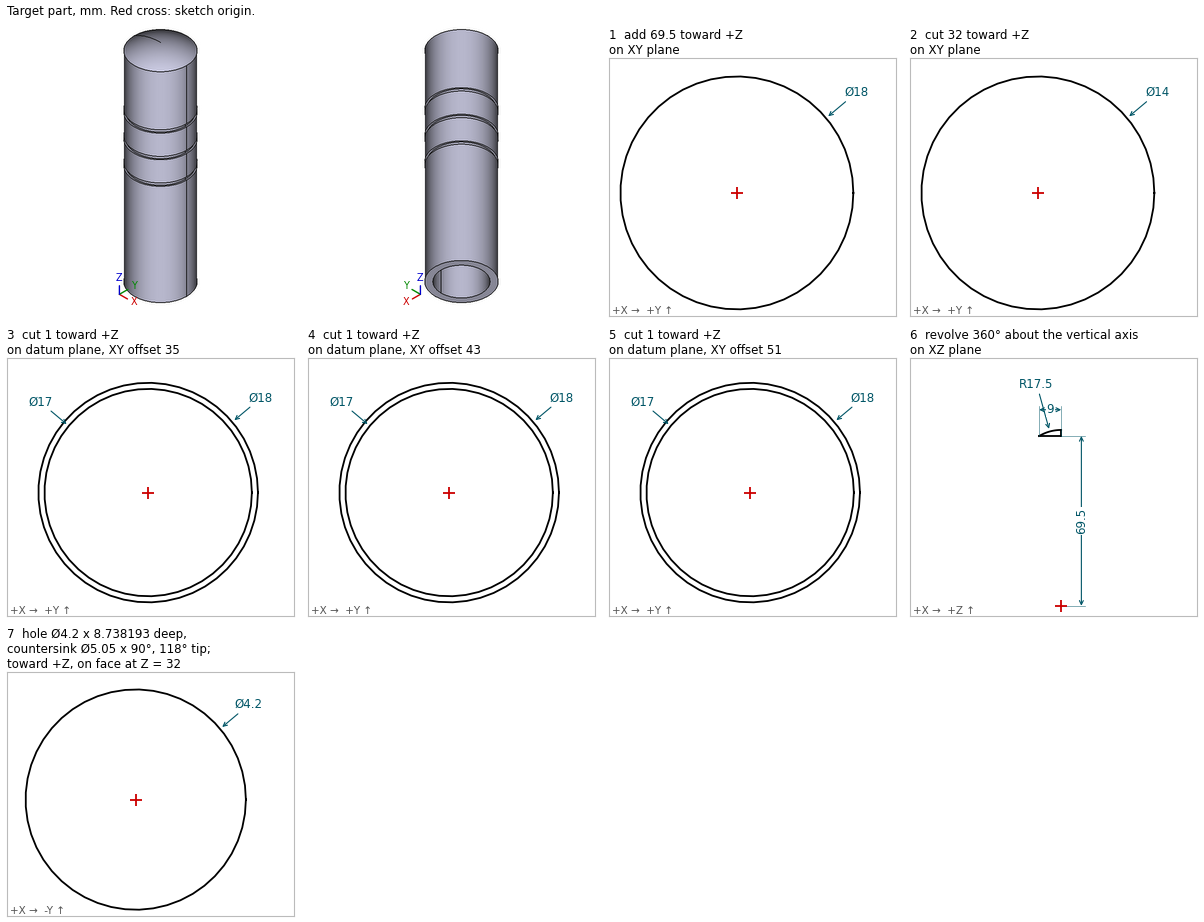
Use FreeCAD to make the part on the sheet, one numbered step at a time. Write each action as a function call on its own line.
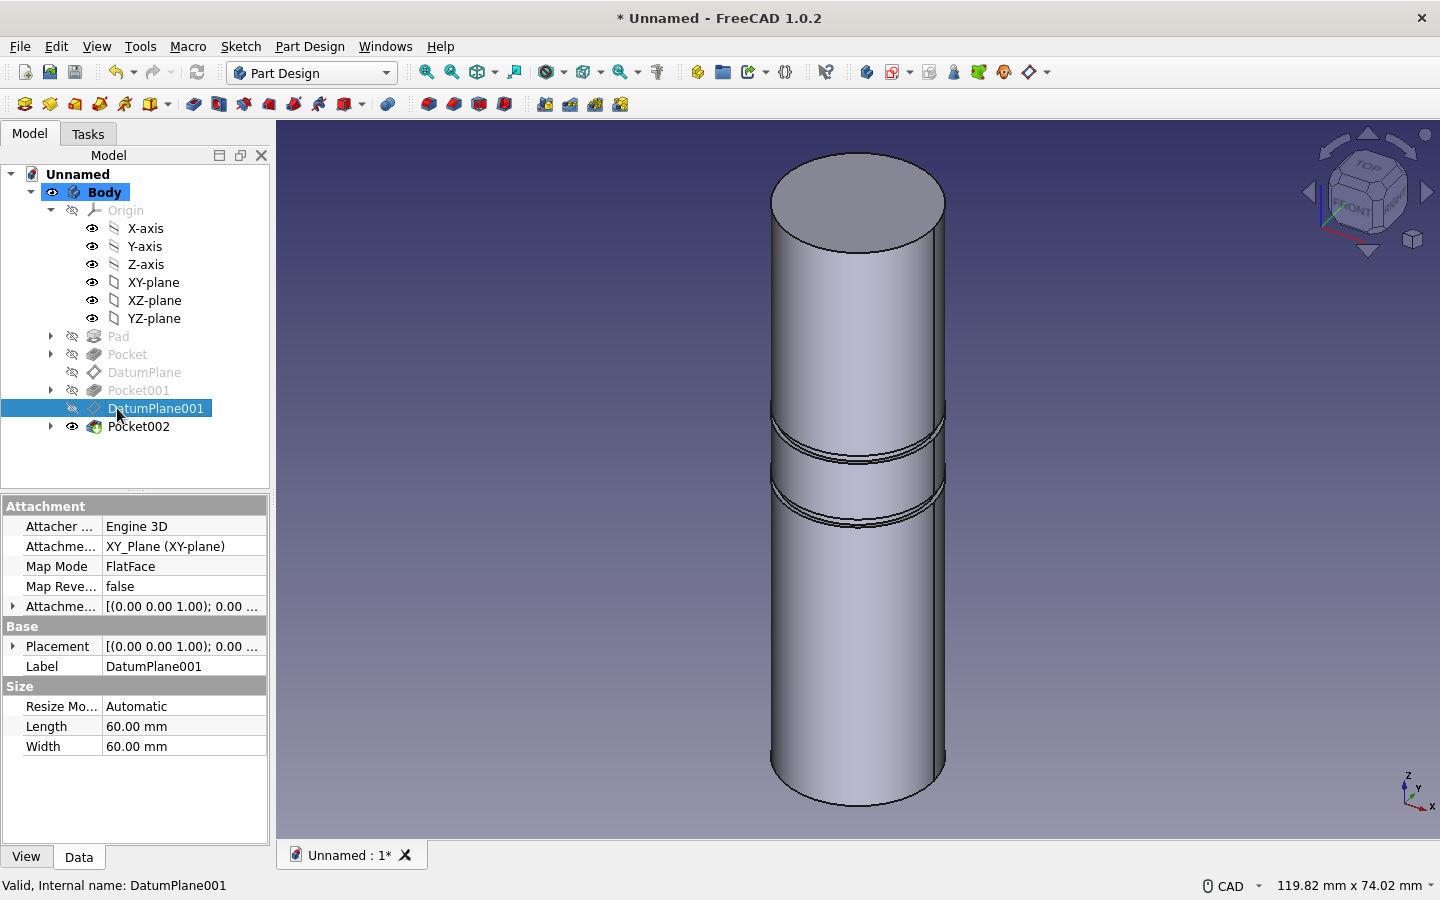
click(137, 282)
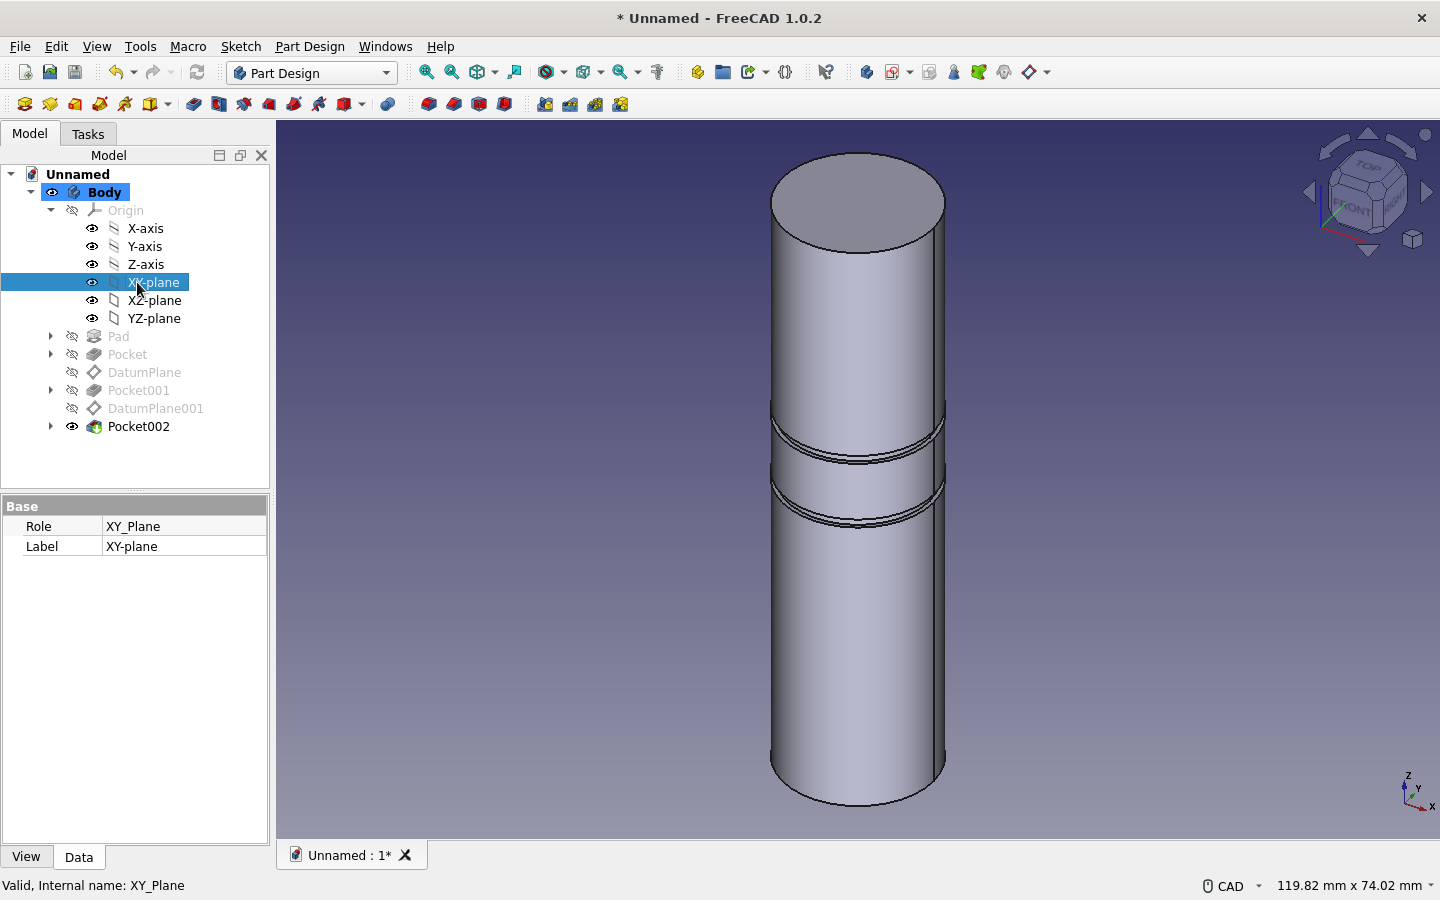
click(1028, 72)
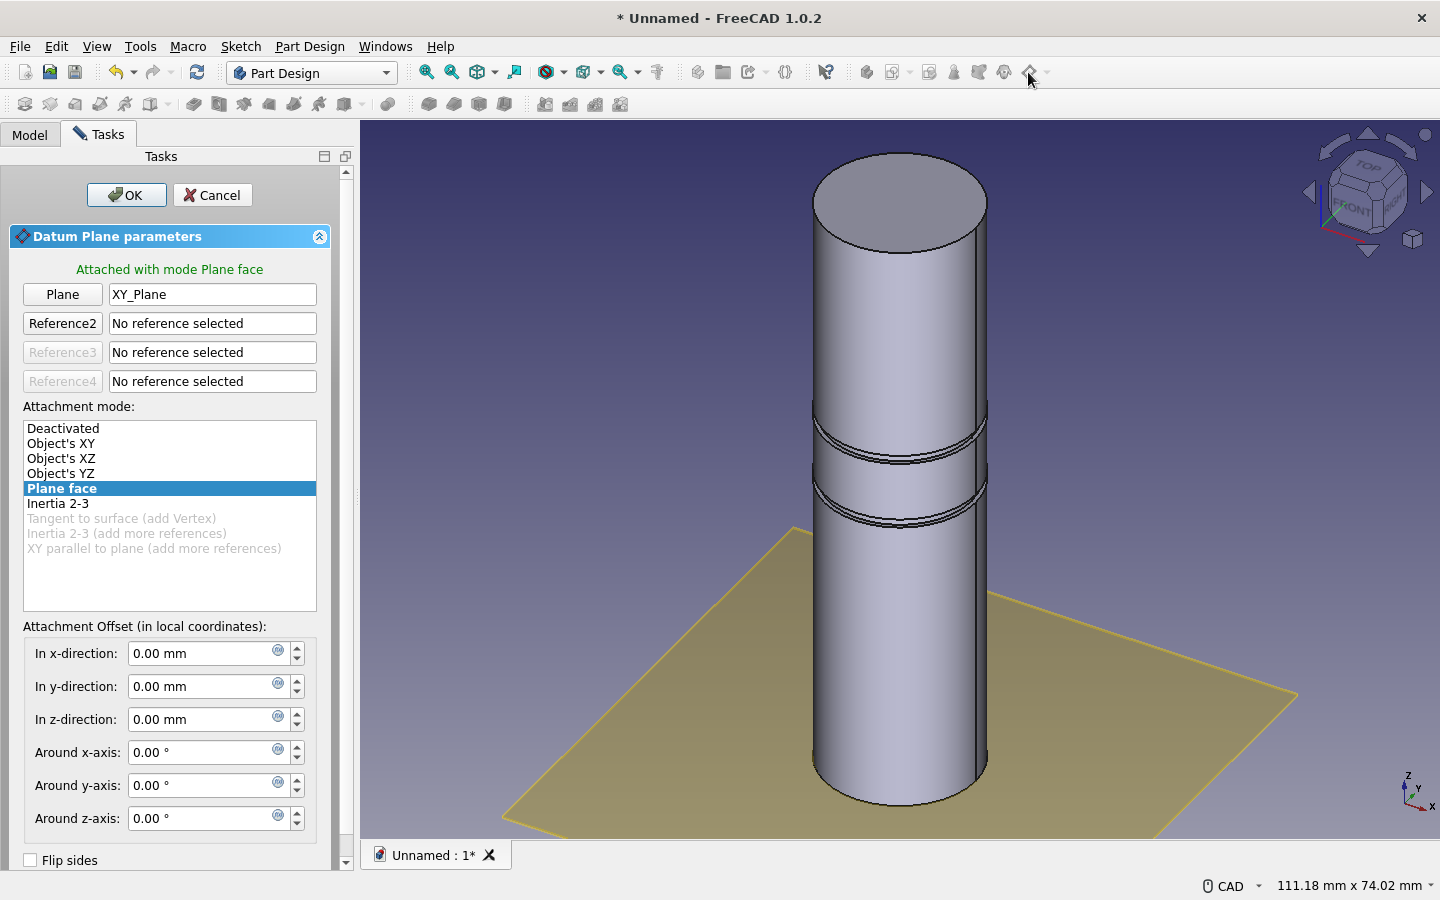
triple_click(210, 720)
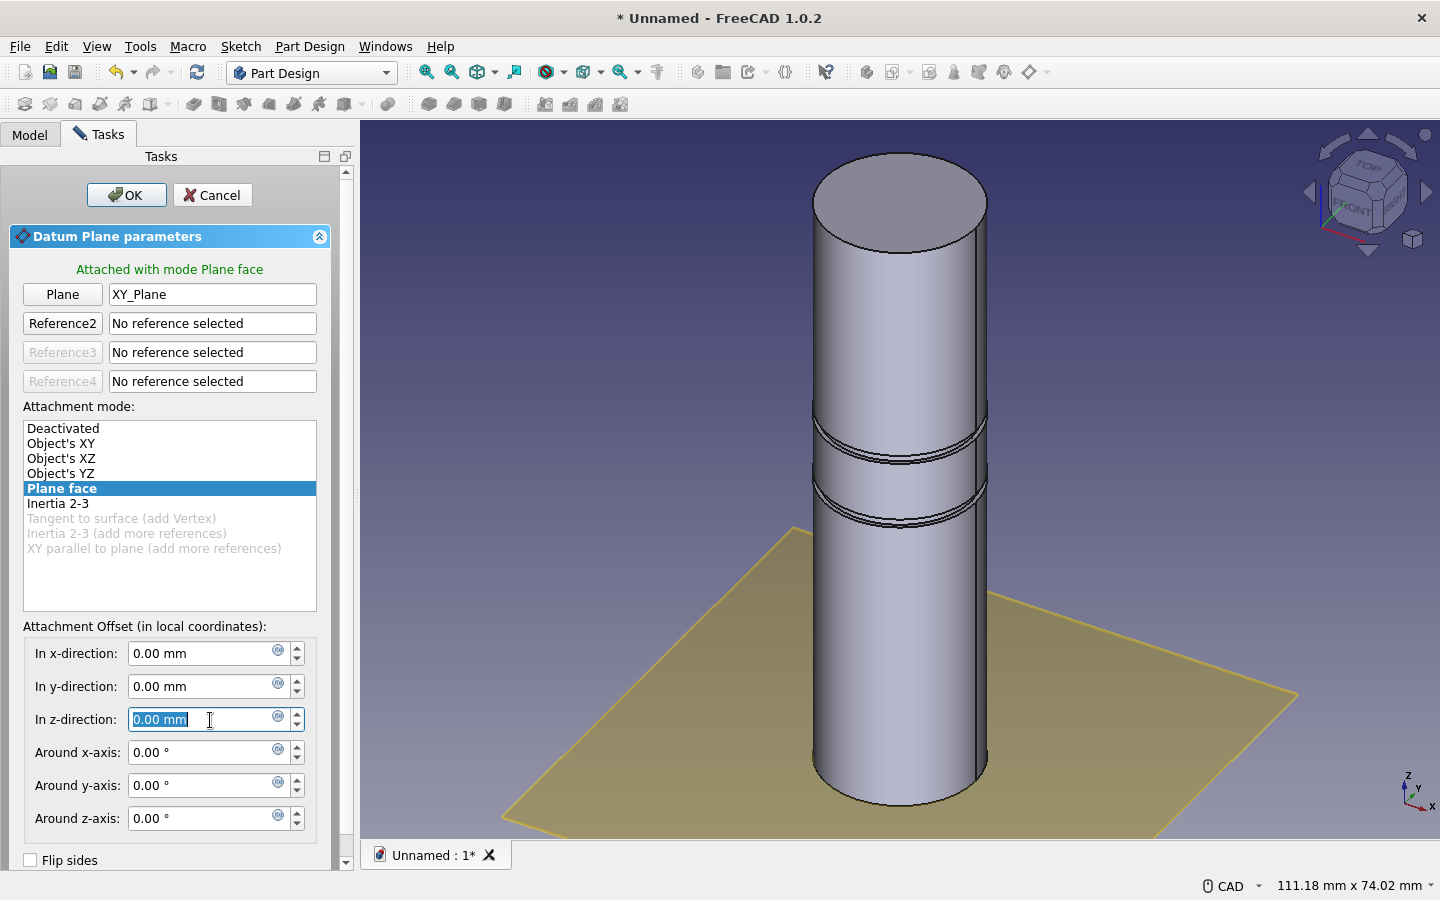
text(51)
key(Tab)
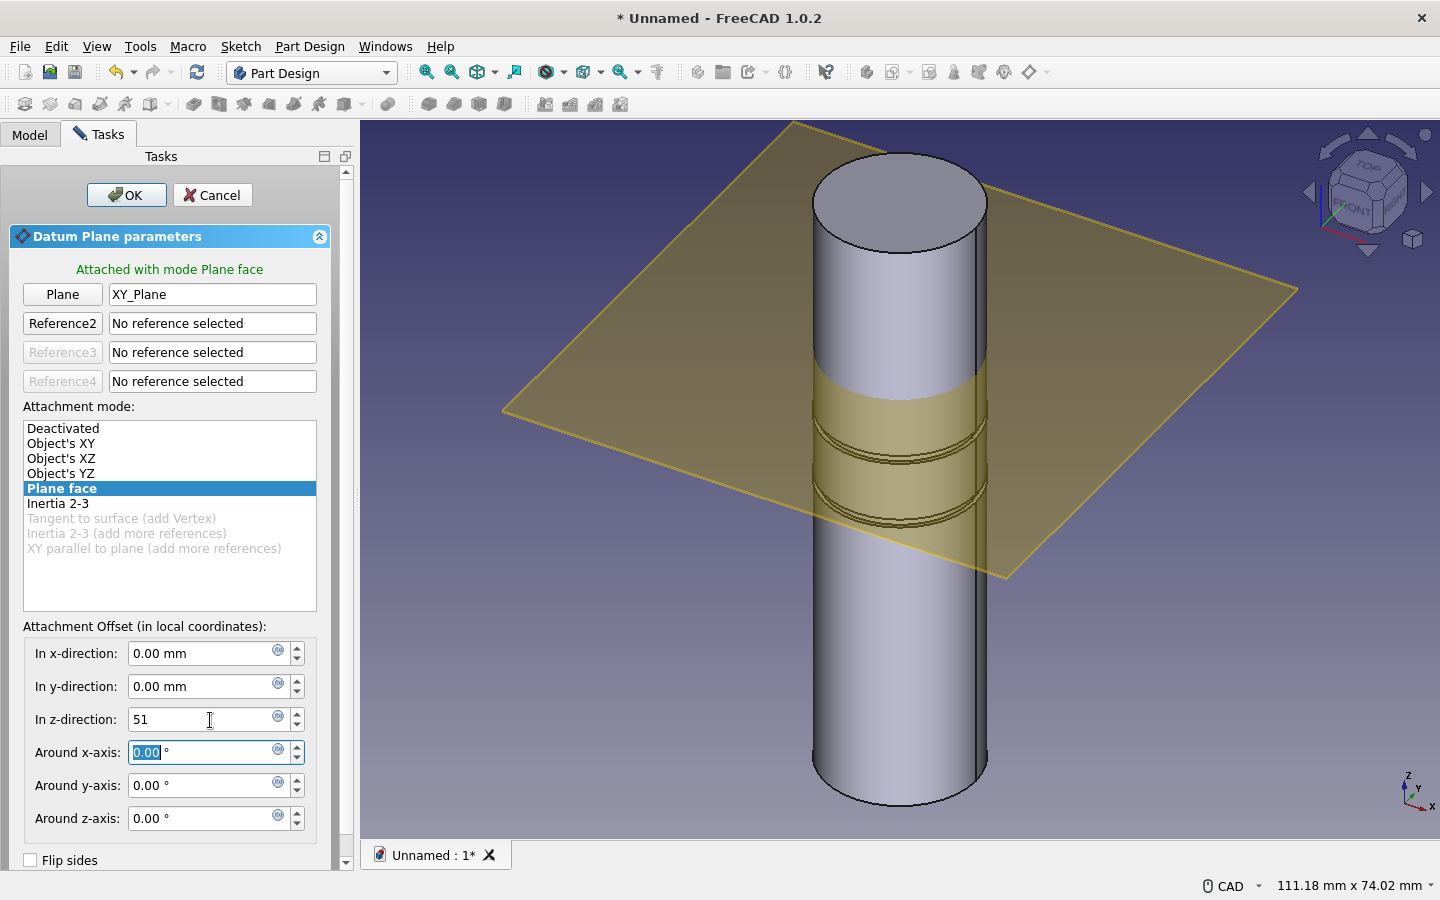
click(127, 195)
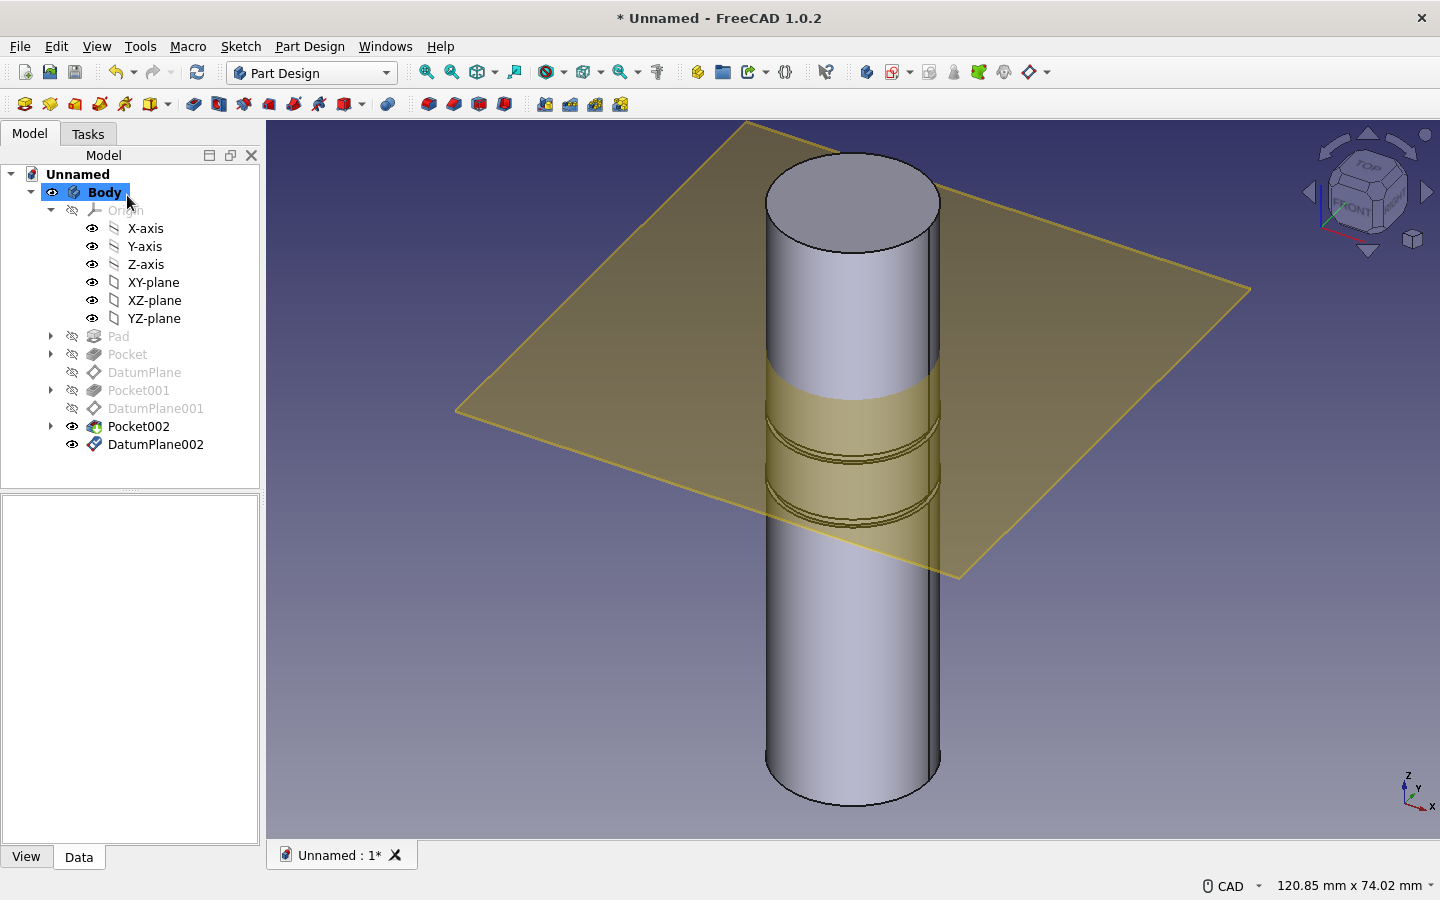
click(117, 444)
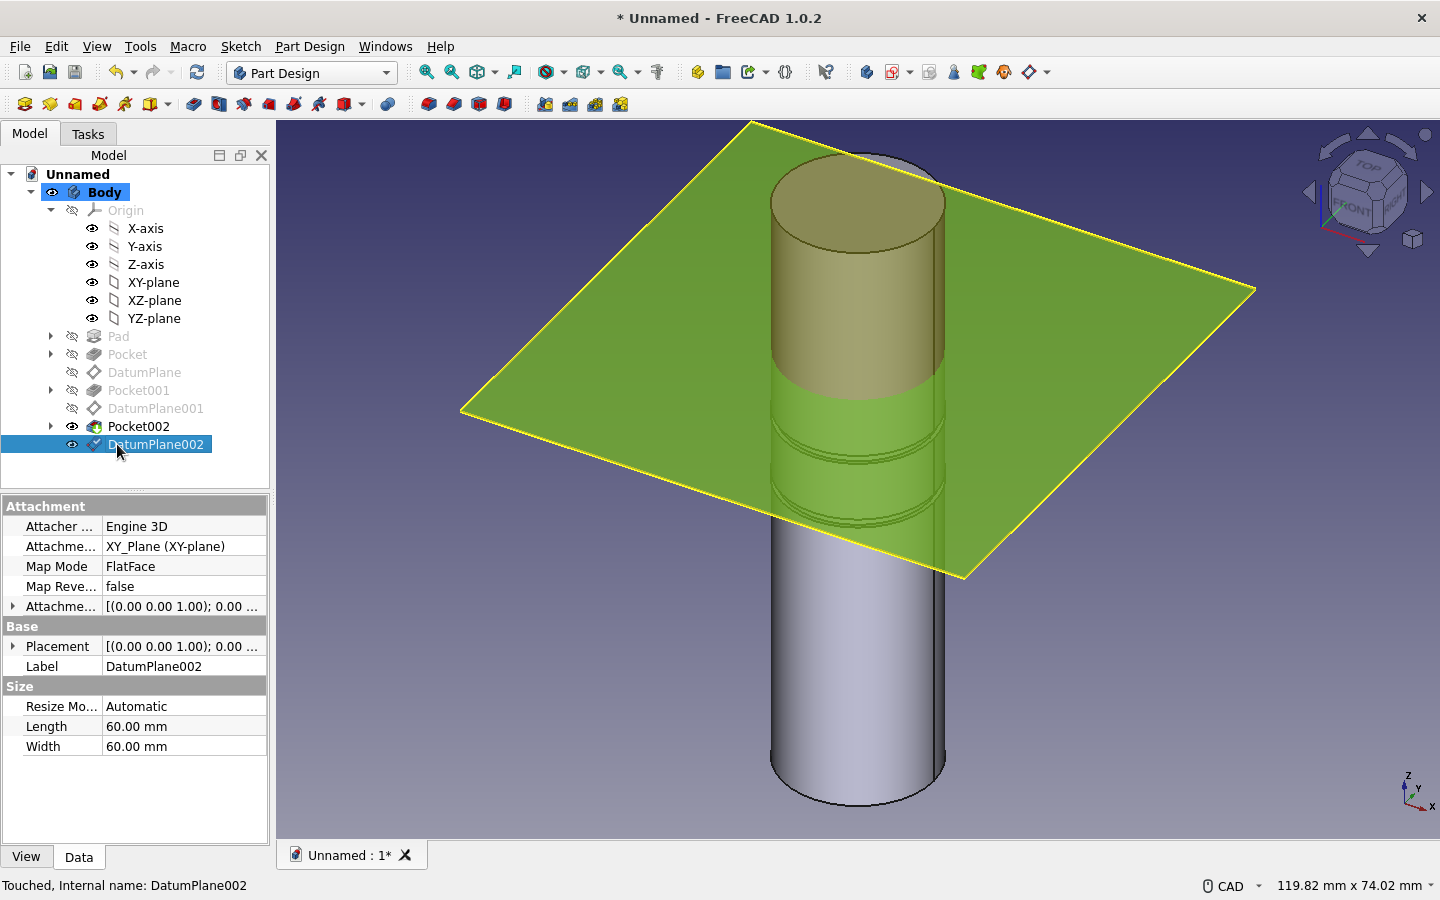
click(892, 72)